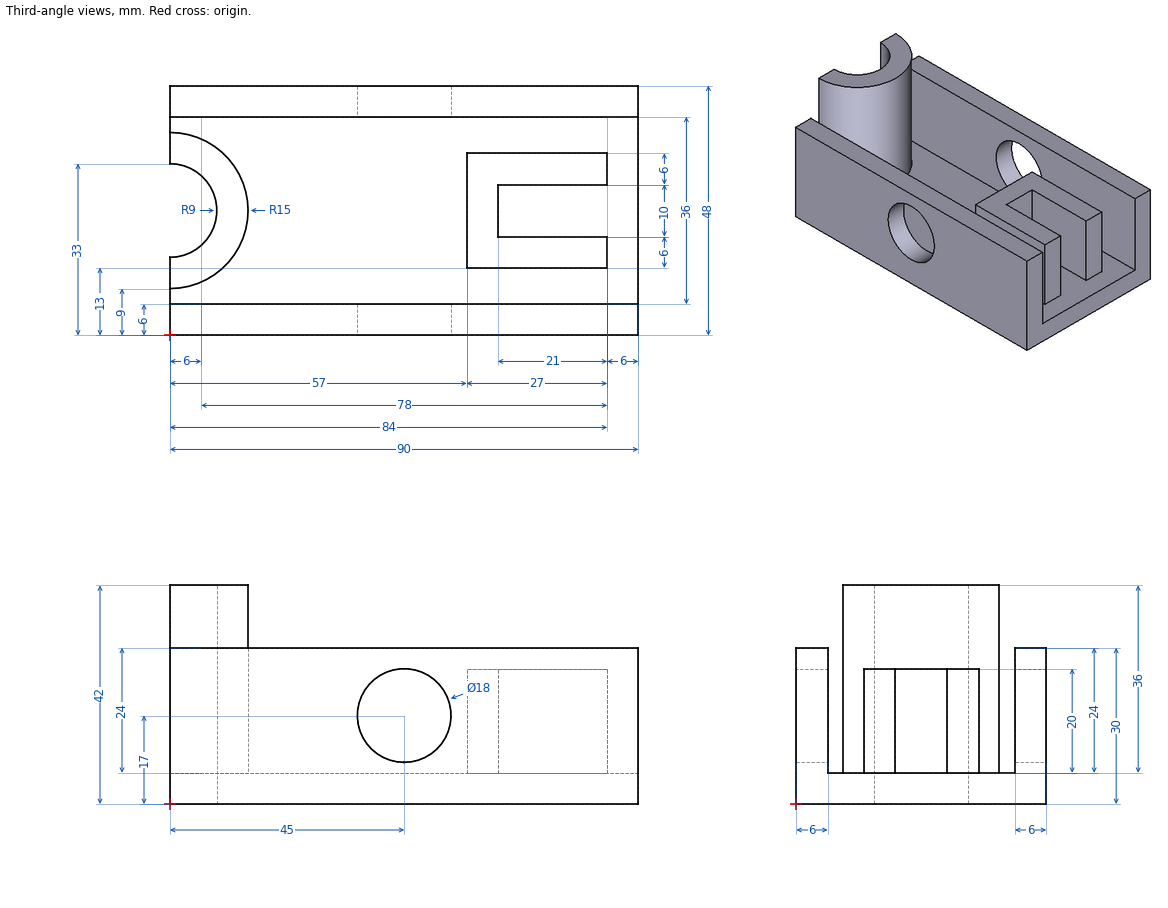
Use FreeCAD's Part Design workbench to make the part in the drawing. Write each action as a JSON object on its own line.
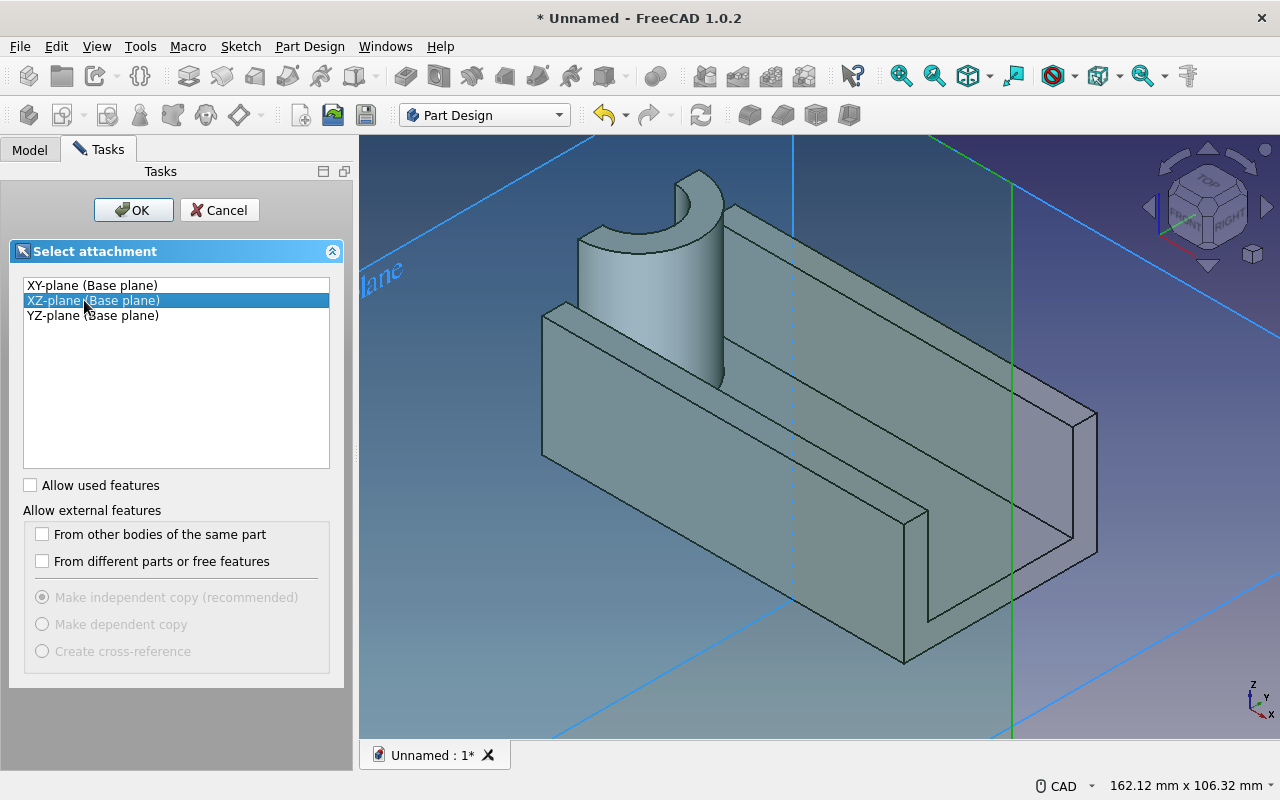
{"action": "left_click", "coordinate": [134, 210]}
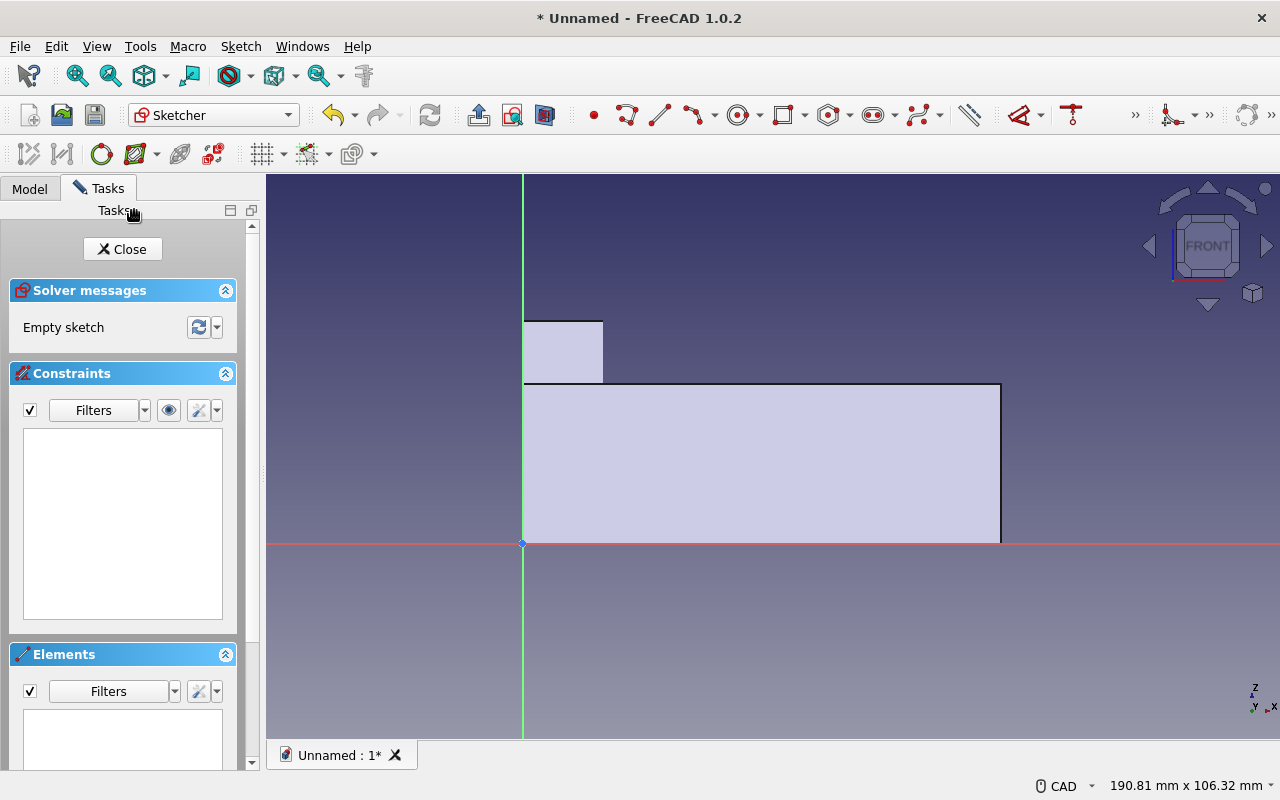
{"action": "scroll", "coordinate": [781, 452], "scroll_direction": "up", "scroll_amount": 7}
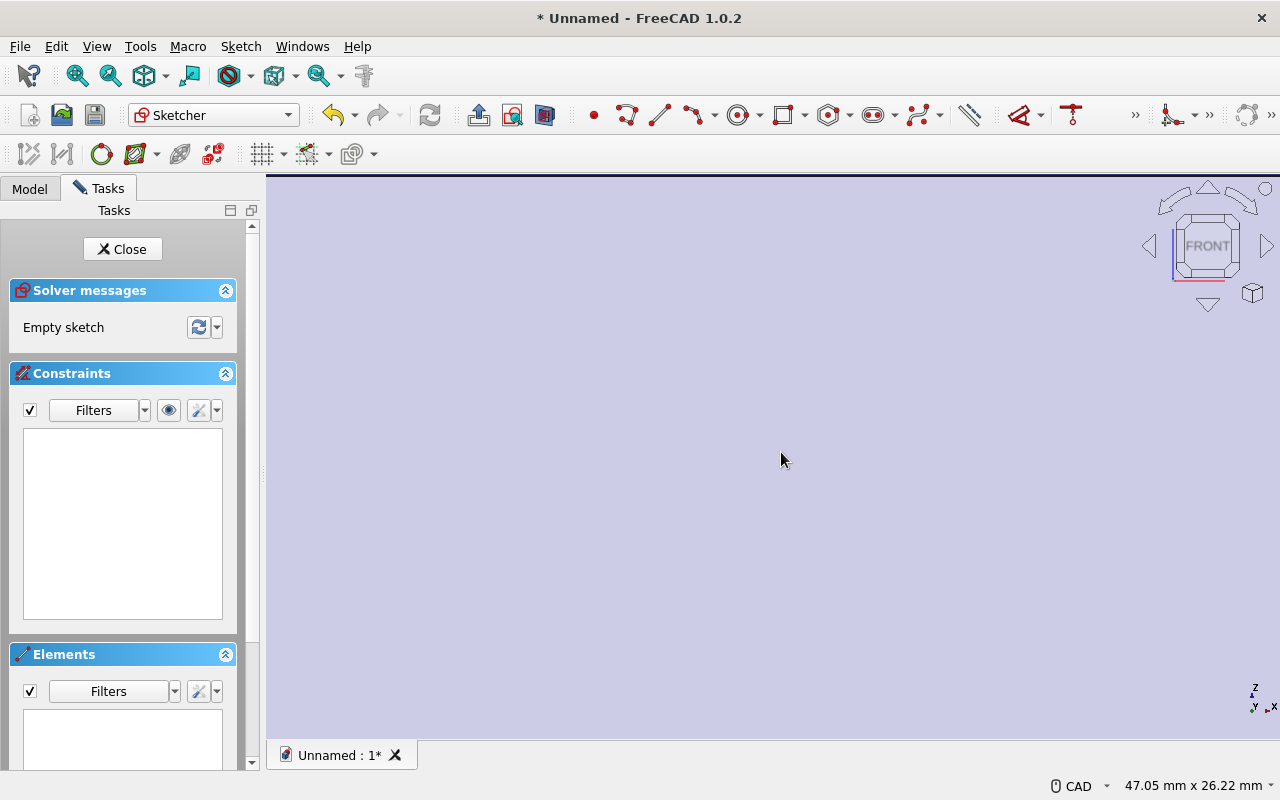
{"action": "left_click", "coordinate": [738, 116]}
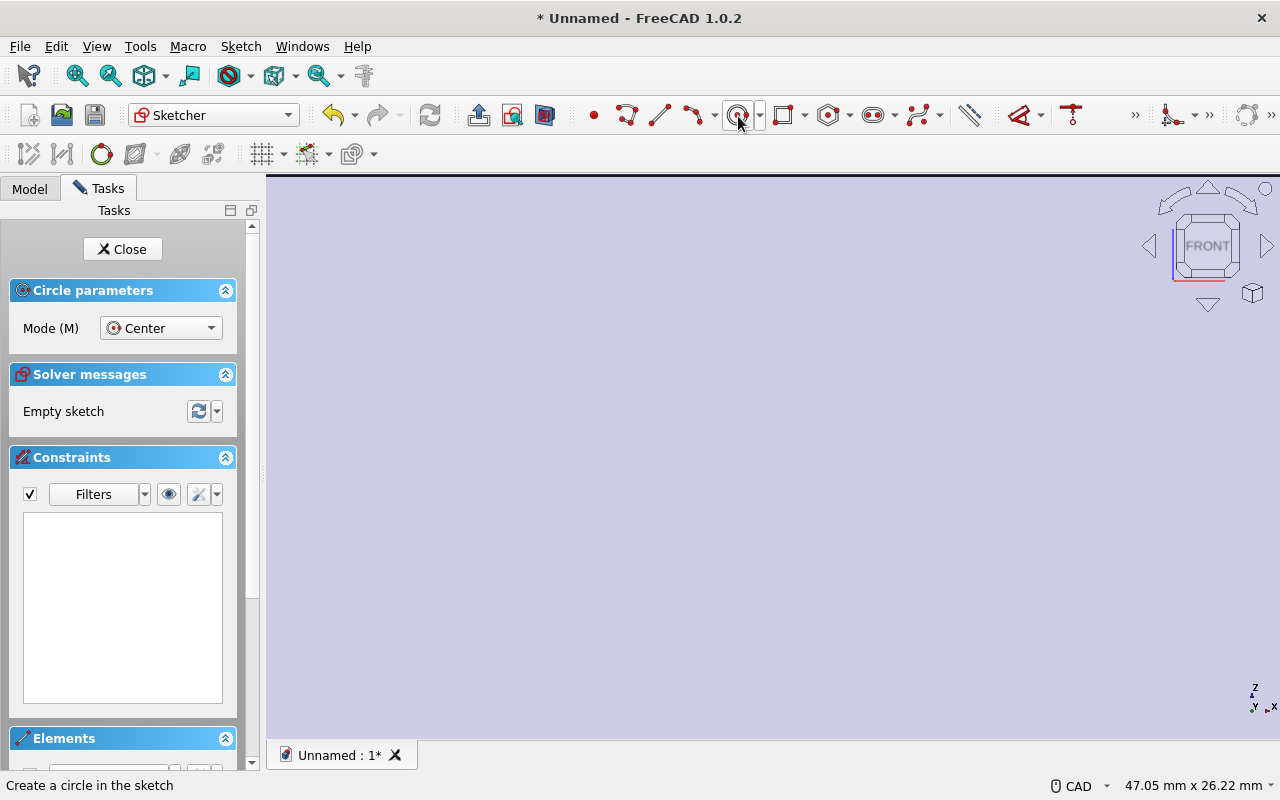
{"action": "left_click", "coordinate": [703, 456]}
{"action": "mouse_move", "coordinate": [840, 319]}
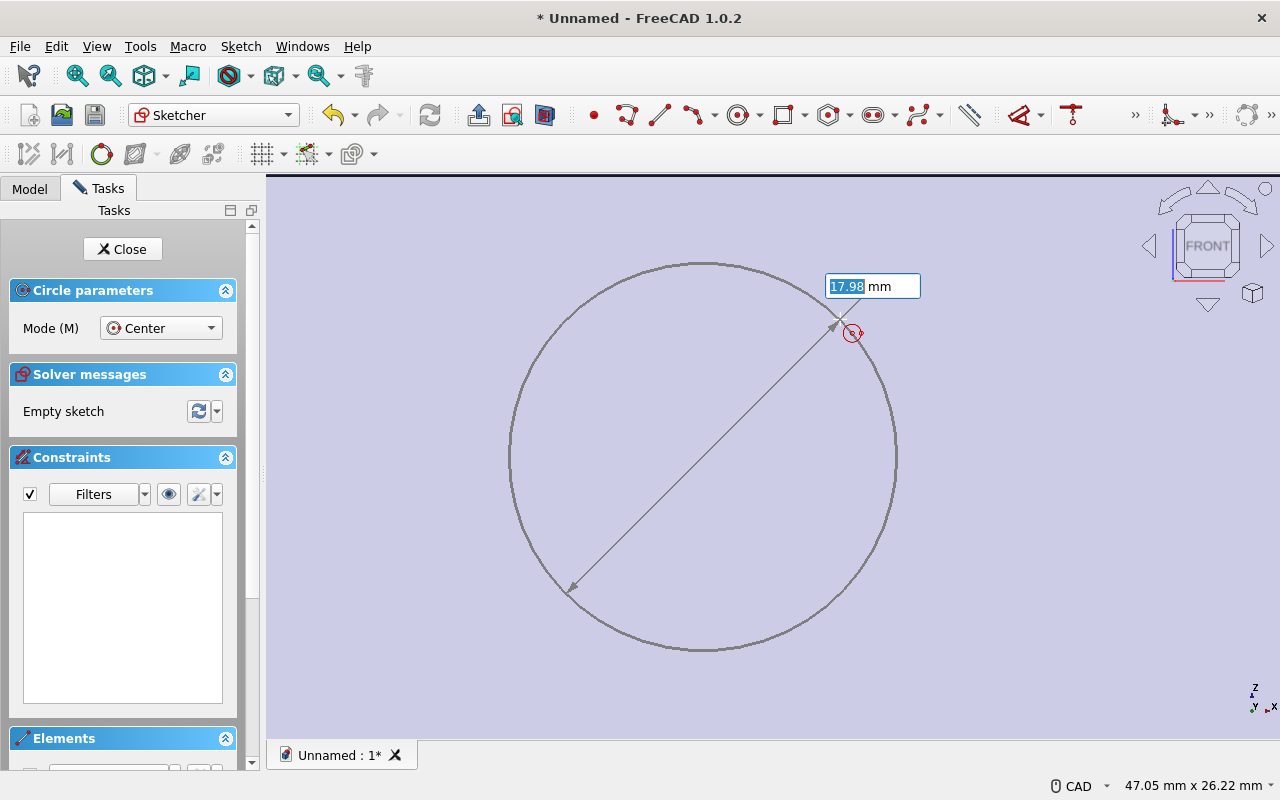
{"action": "type", "text": "18"}
{"action": "key", "text": "Return"}
{"action": "key", "text": "Escape"}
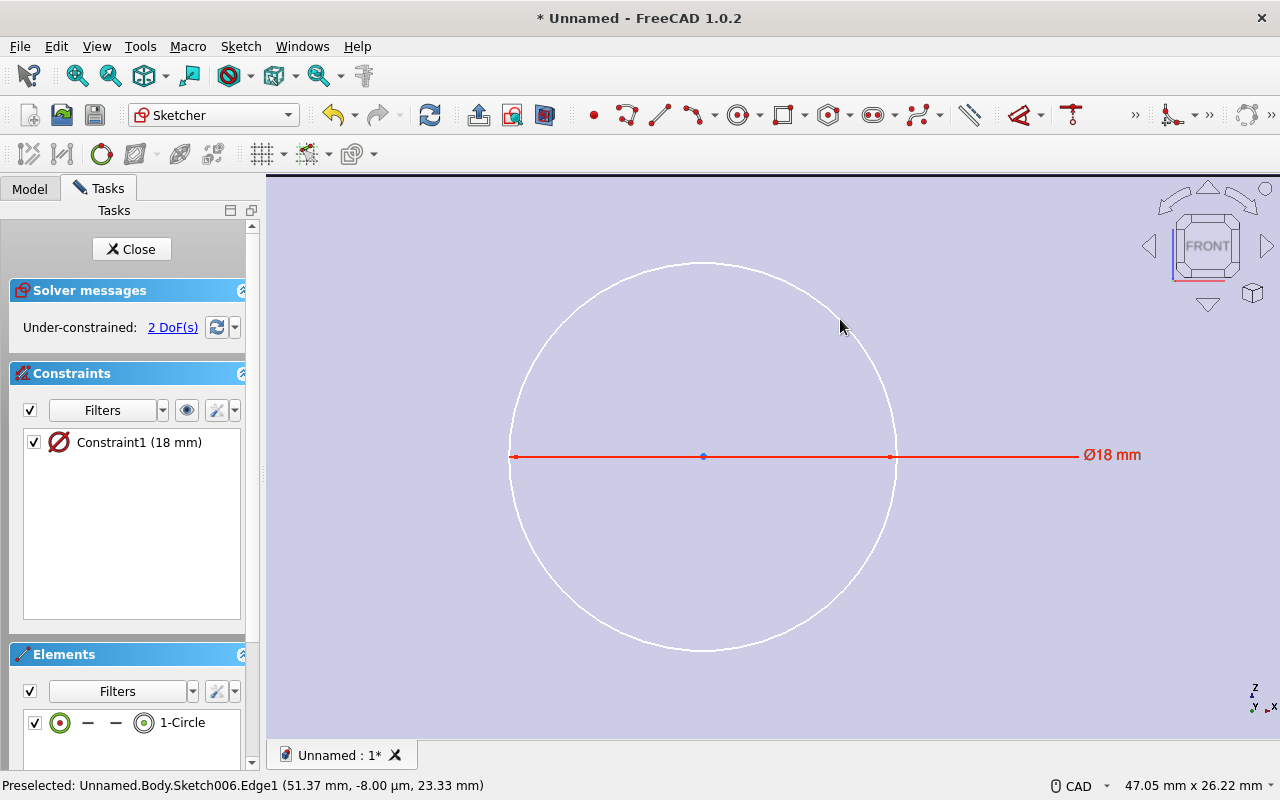
{"action": "key", "text": "d"}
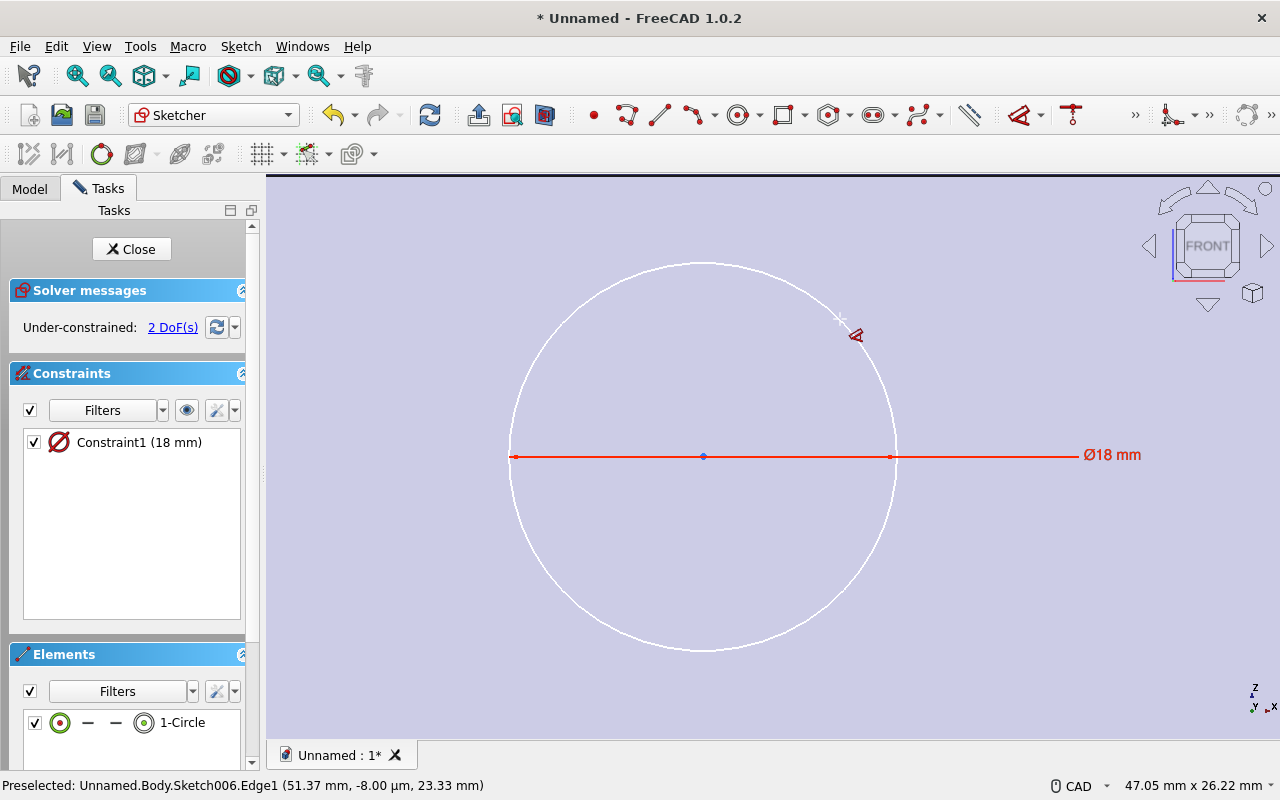
{"action": "left_click", "coordinate": [703, 457]}
{"action": "left_click", "coordinate": [499, 423]}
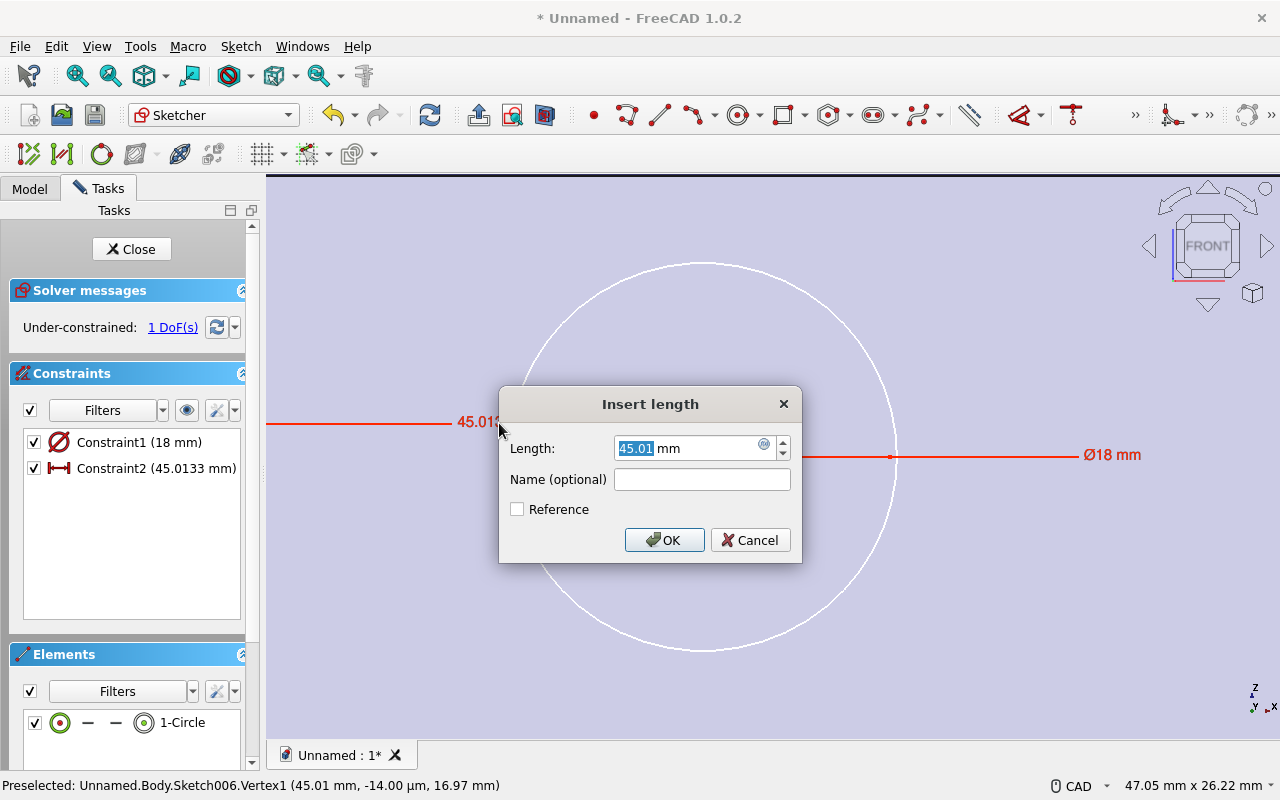
{"action": "type", "text": "45"}
{"action": "key", "text": "Return"}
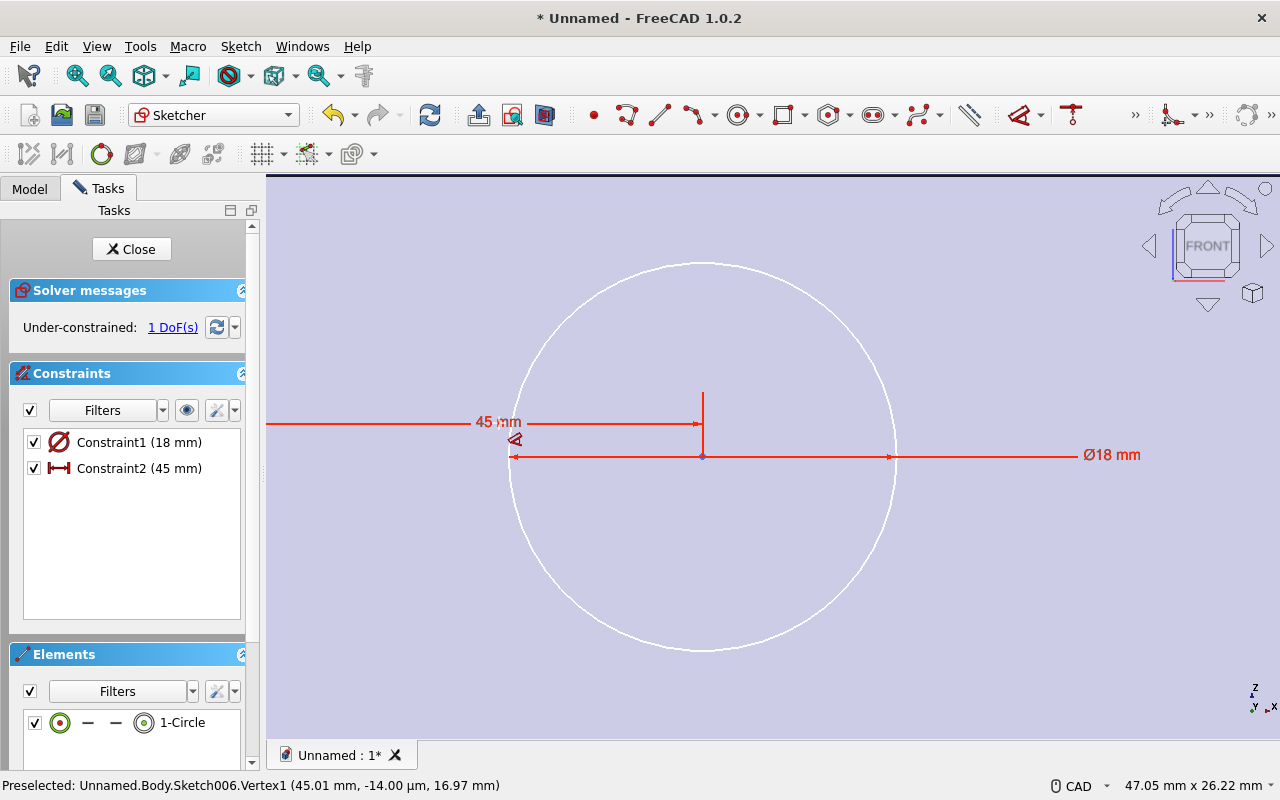
{"action": "left_click", "coordinate": [703, 457]}
{"action": "left_click", "coordinate": [737, 584]}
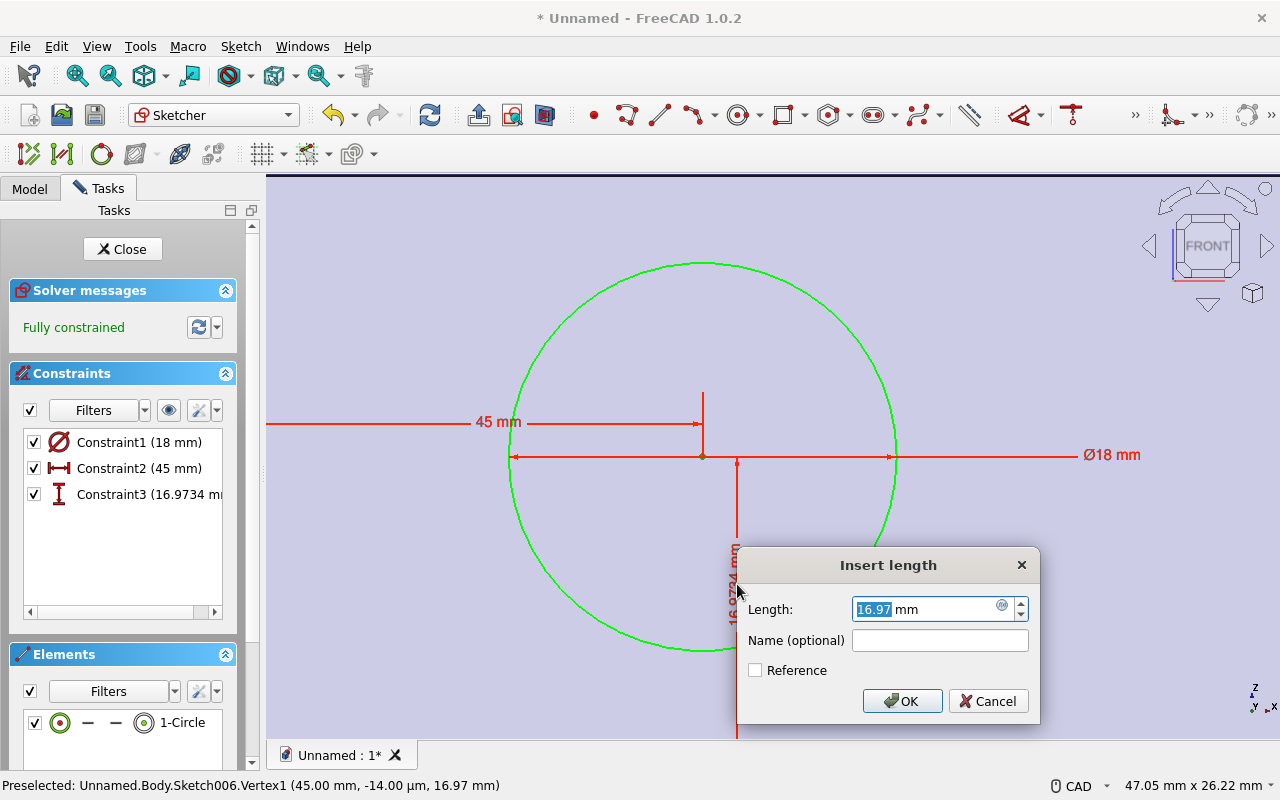
{"action": "type", "text": "17"}
{"action": "key", "text": "Return"}
{"action": "key", "text": "Escape"}